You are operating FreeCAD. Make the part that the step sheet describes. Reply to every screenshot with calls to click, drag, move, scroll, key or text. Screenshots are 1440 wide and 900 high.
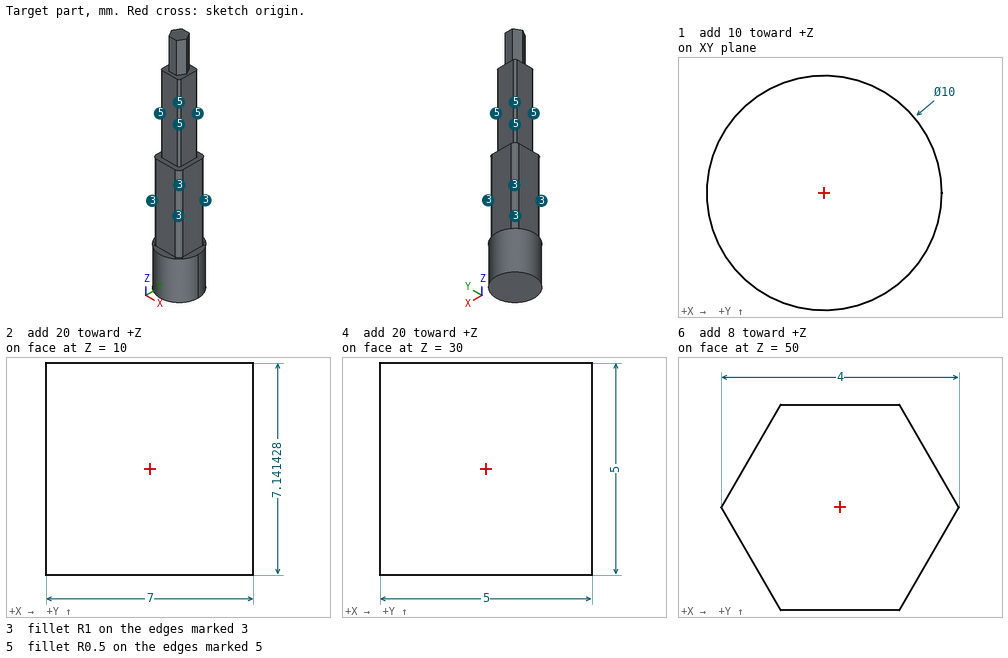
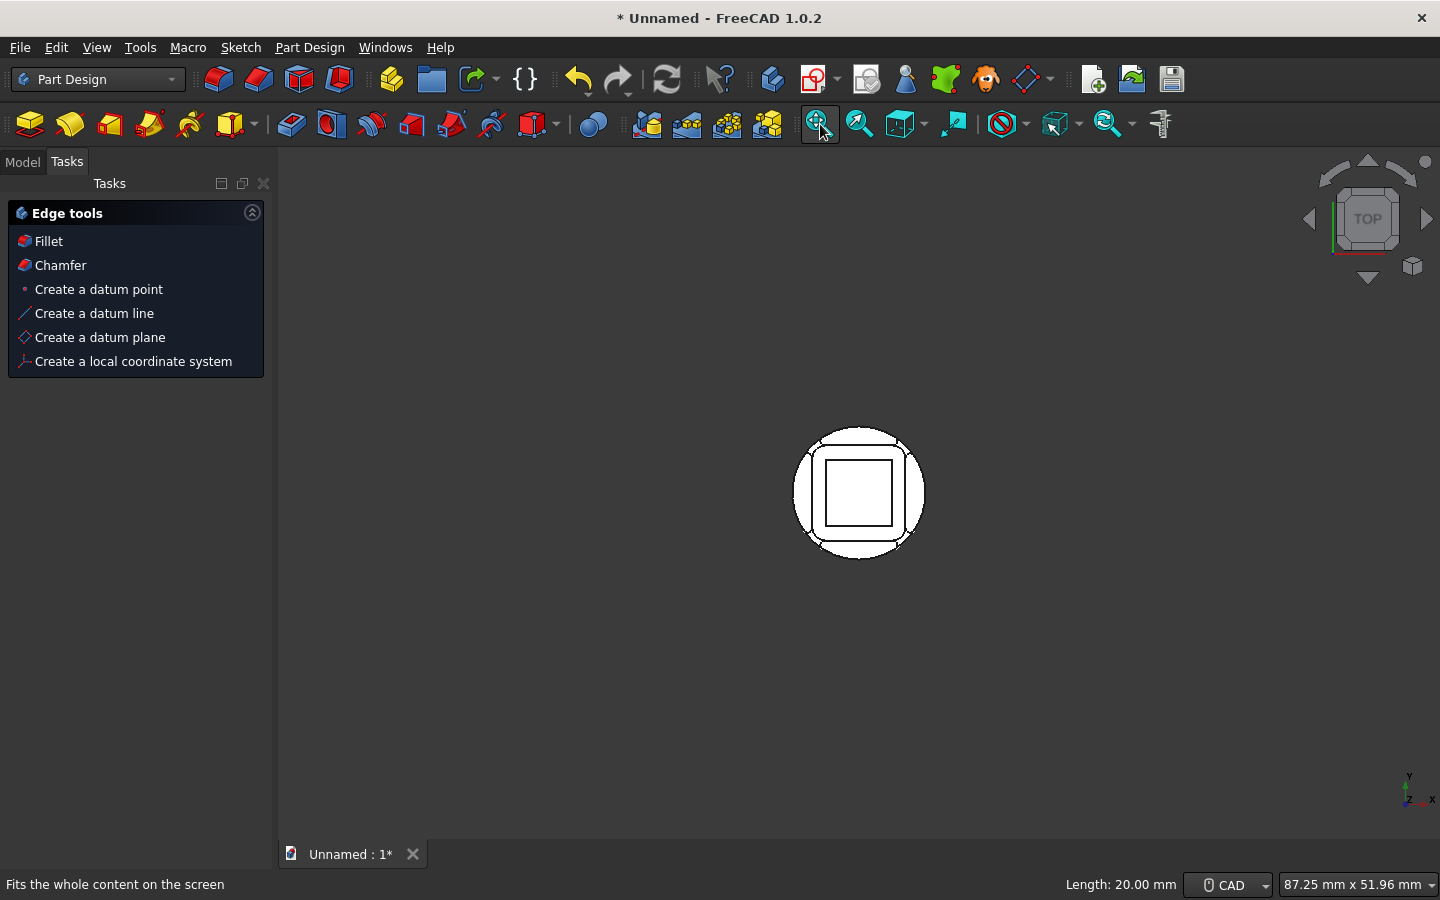
key(0)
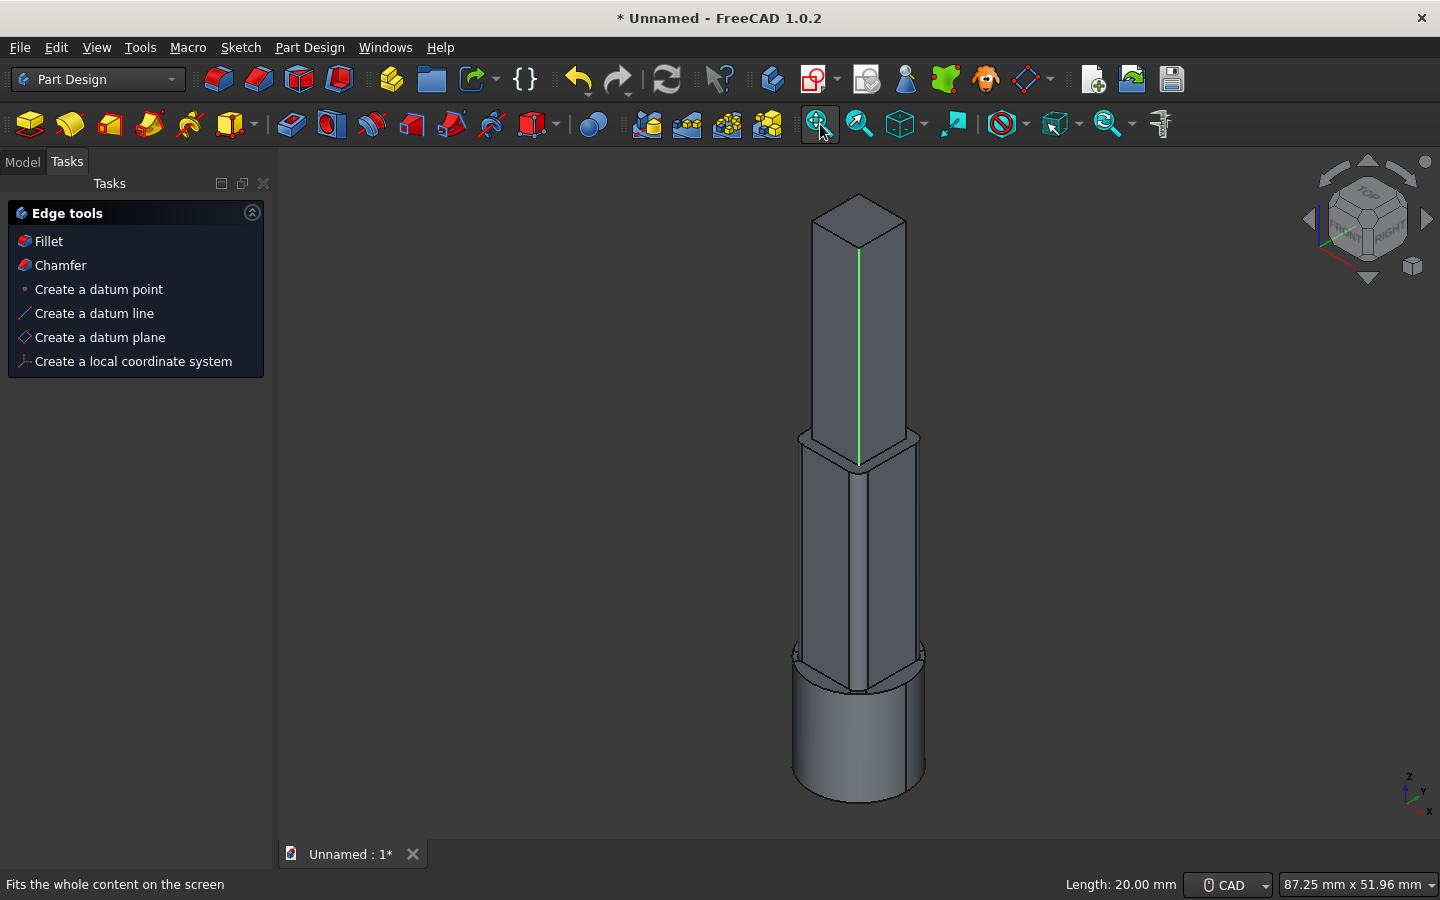
key(1)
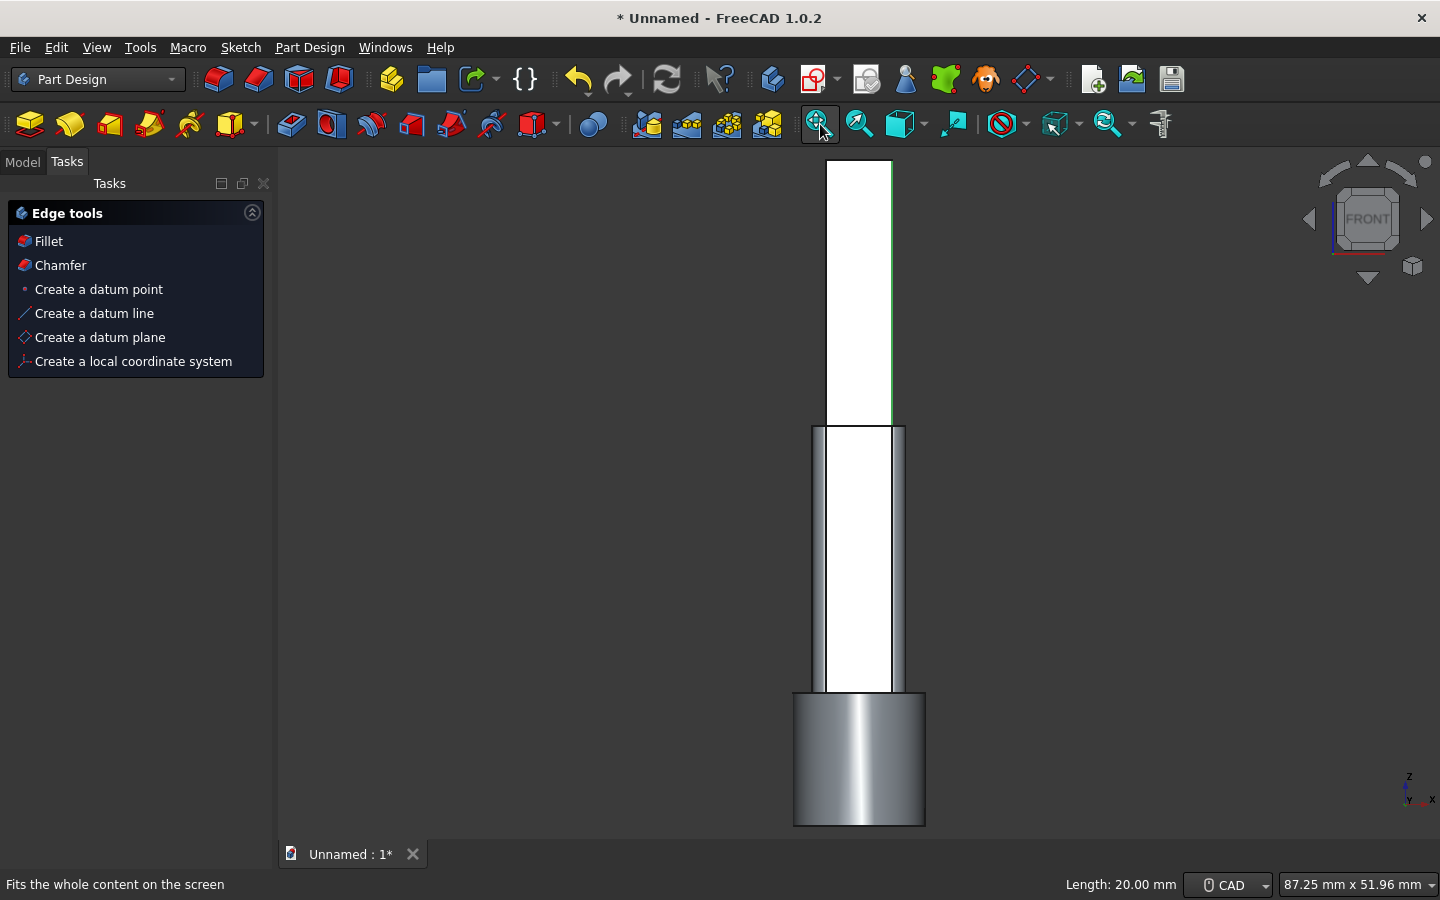
click(826, 292, ctrl)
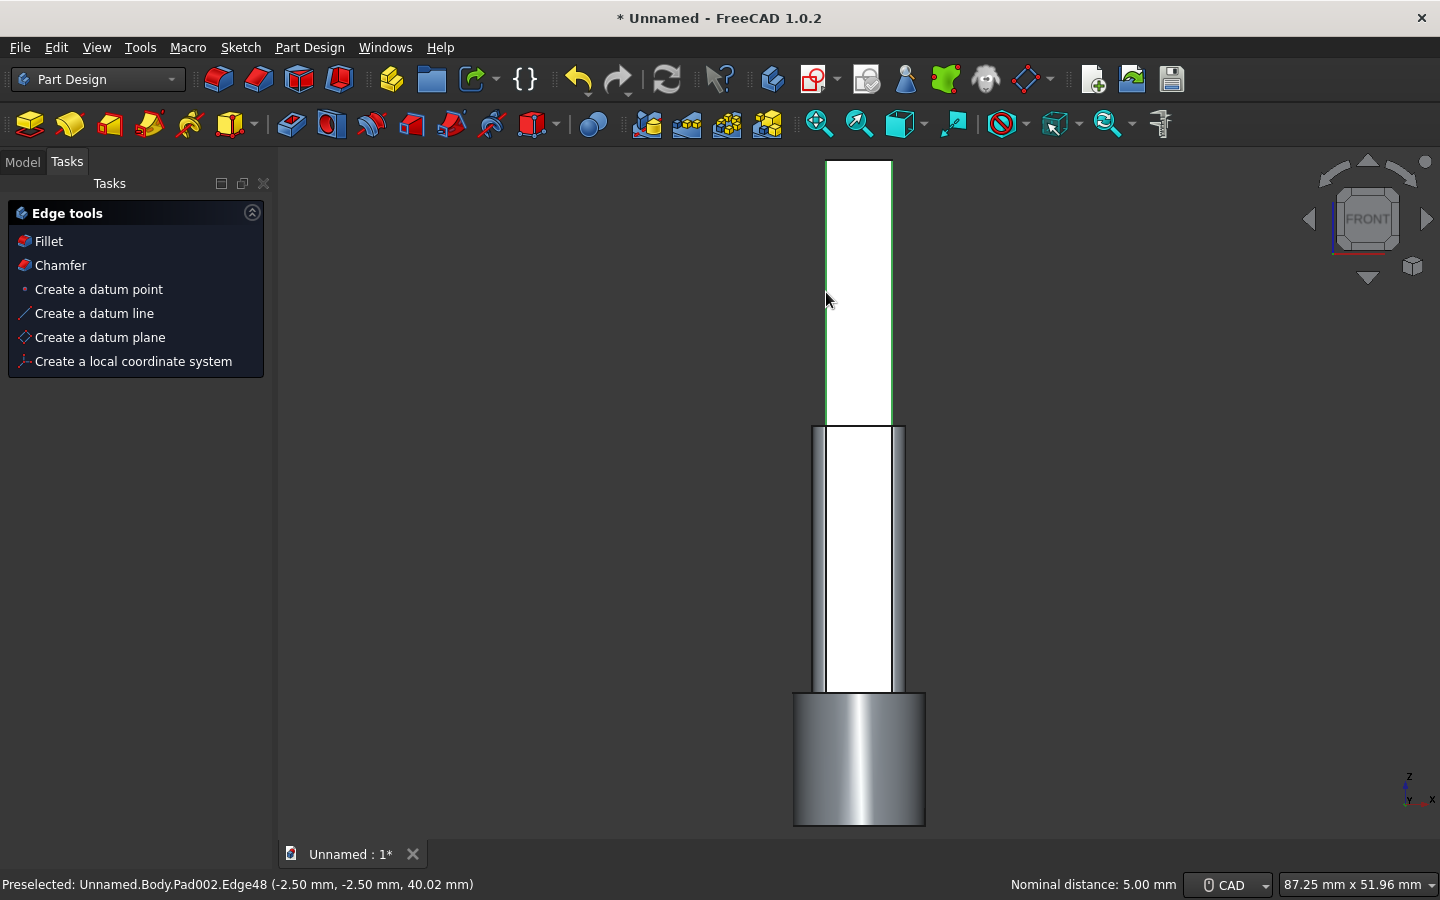
key(3)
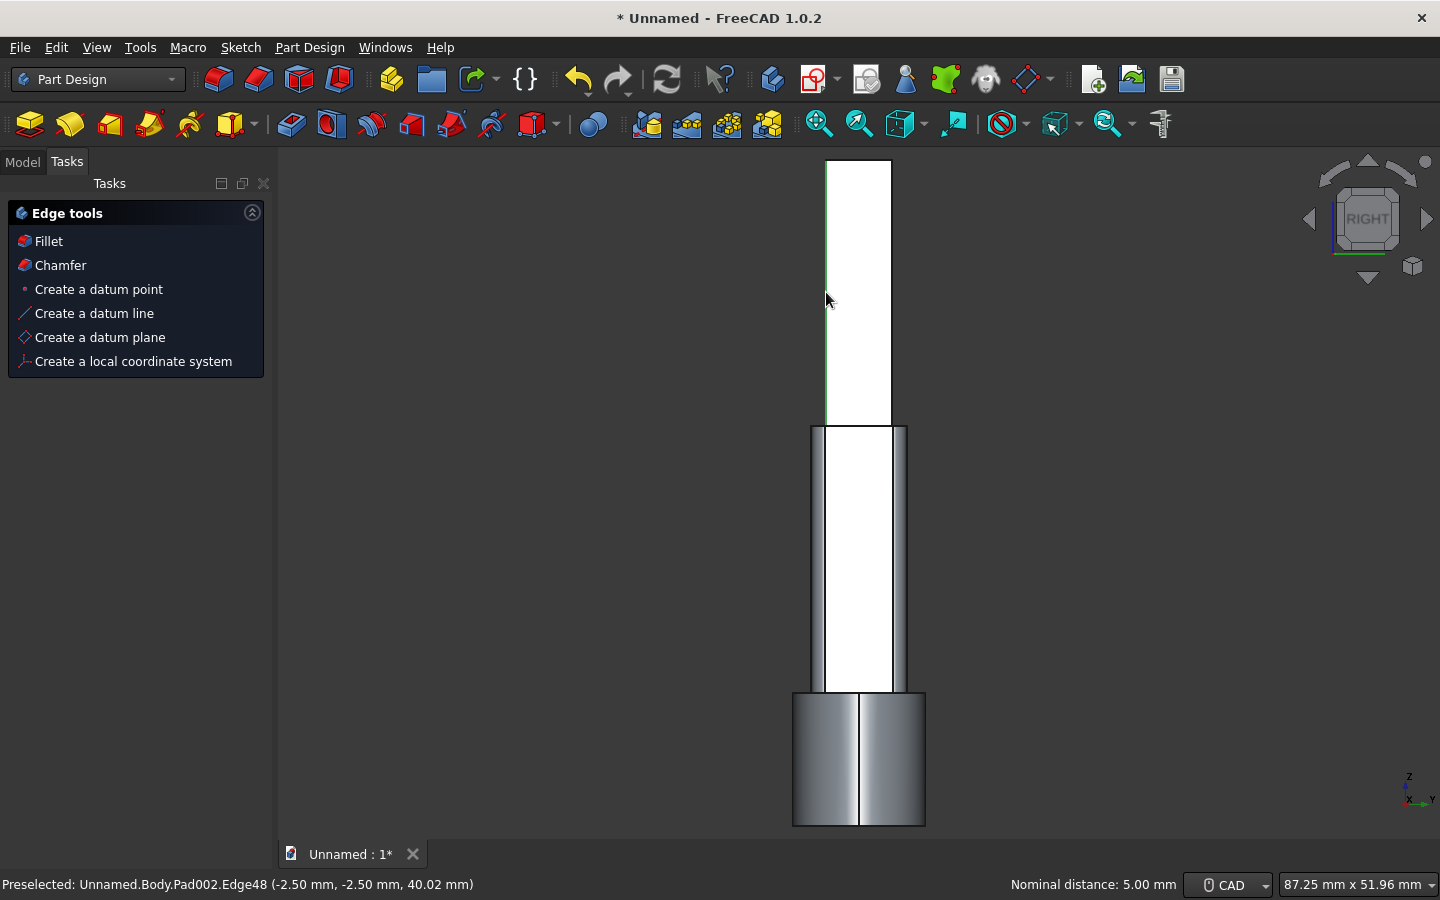
click(892, 292, ctrl)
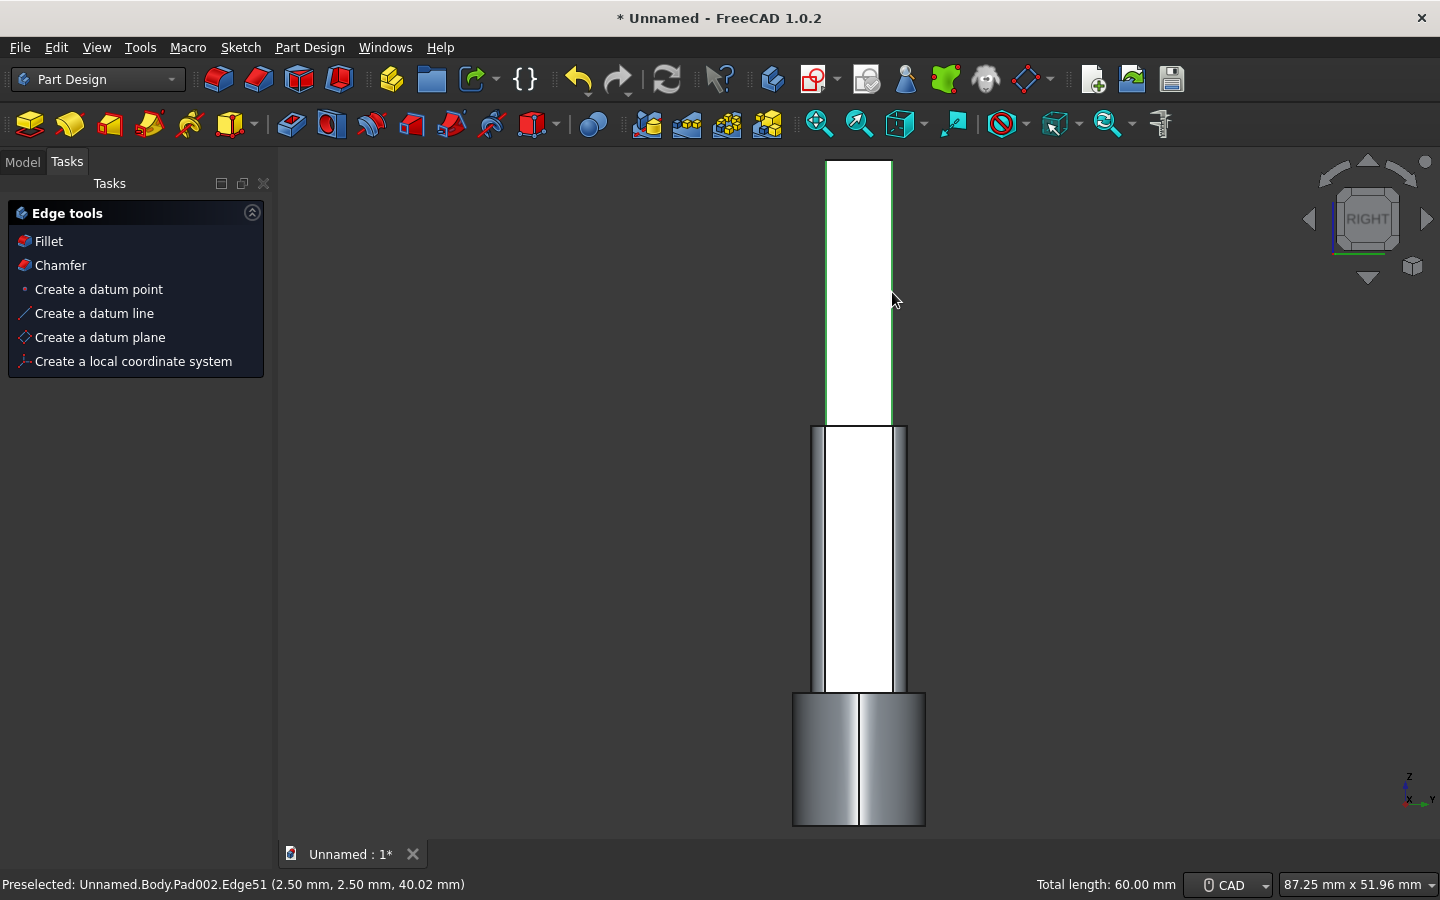
key(5)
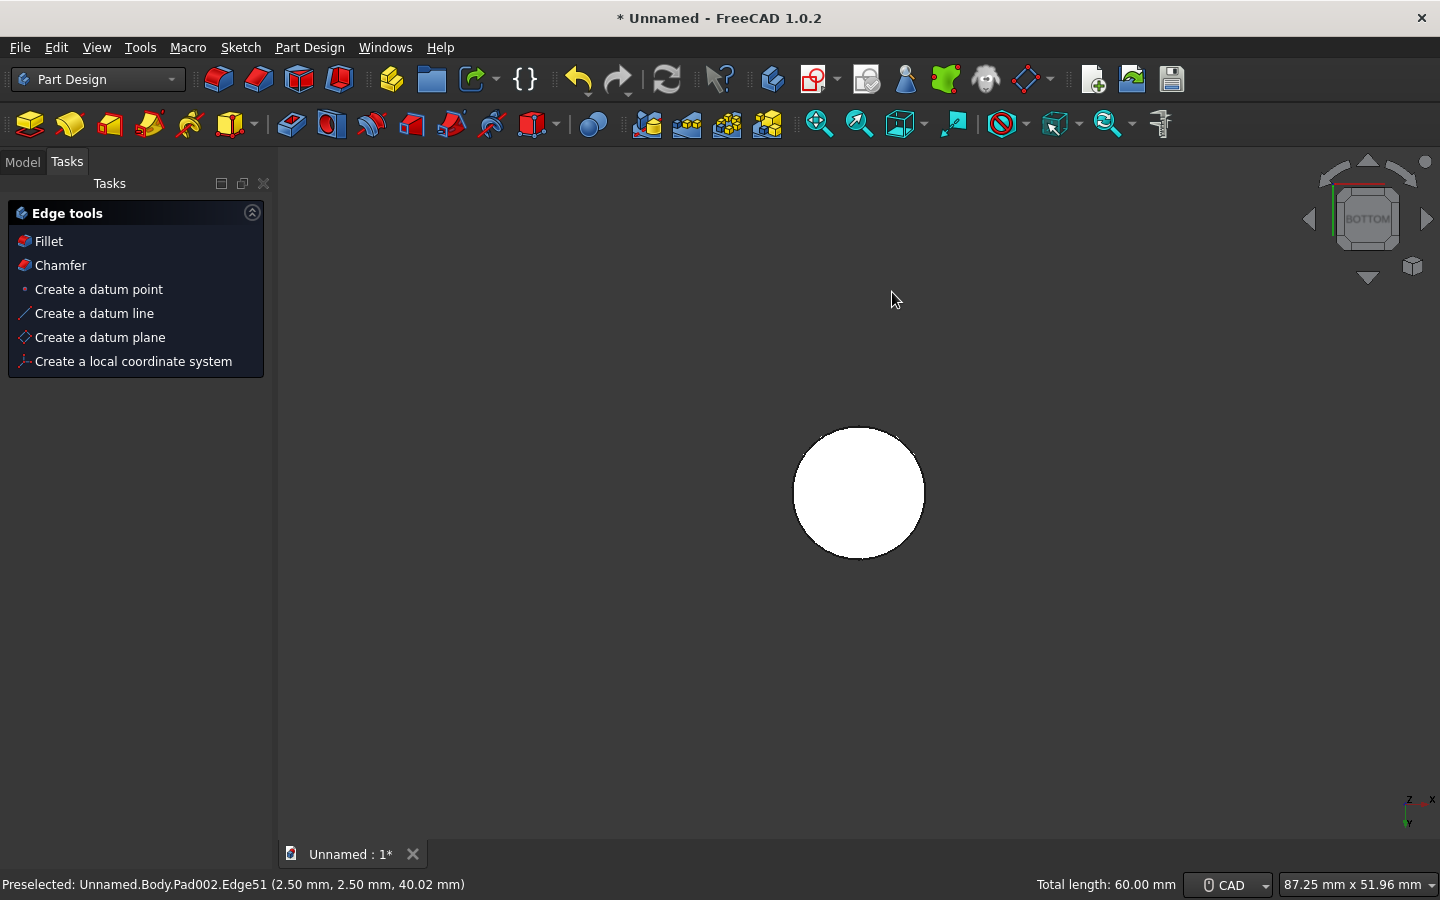
key(v)
key(f)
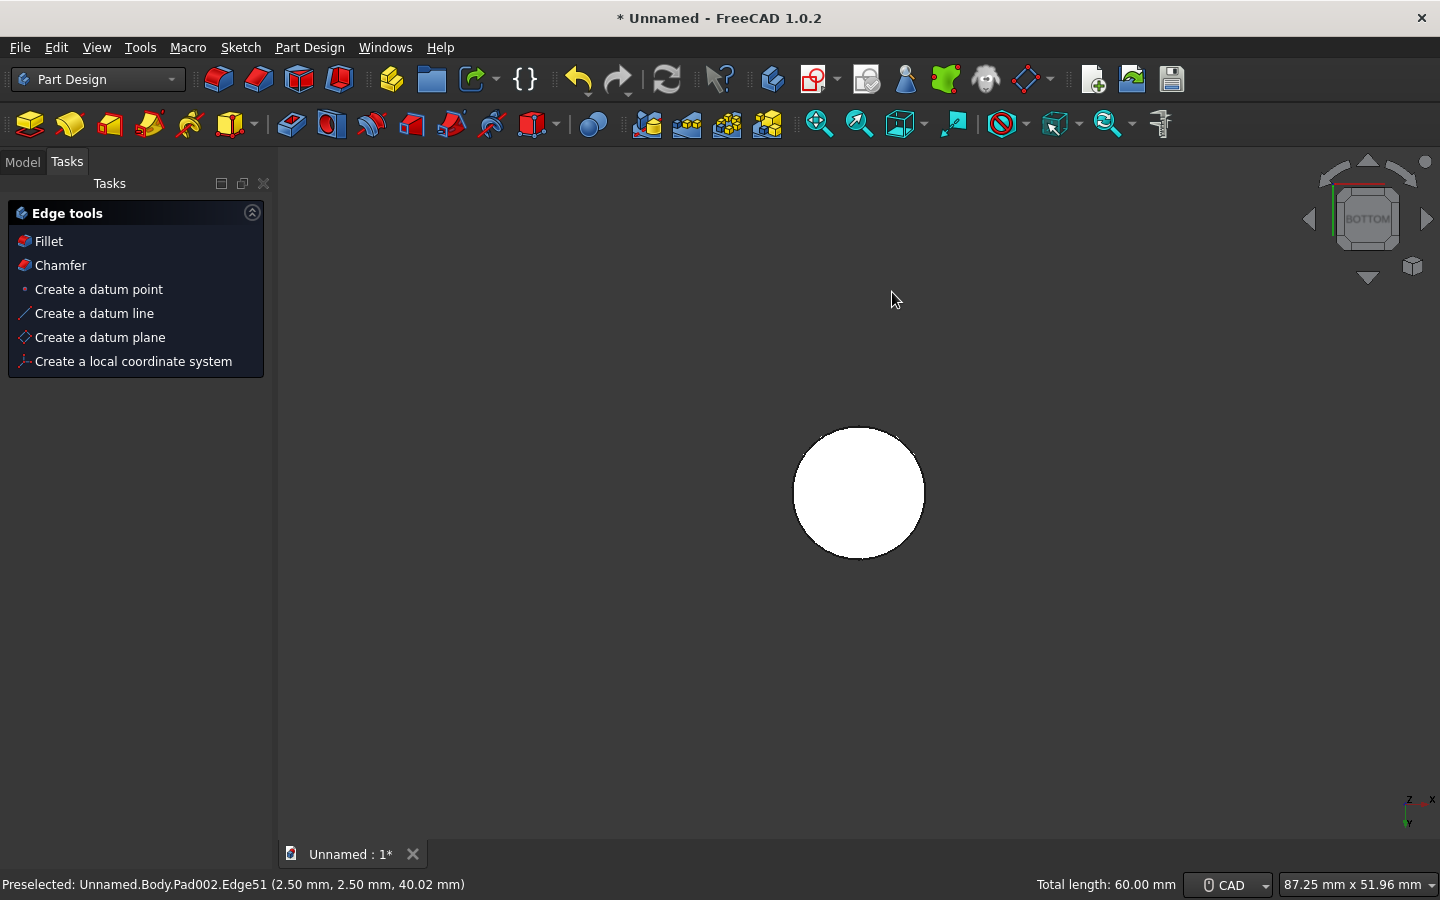
key(4)